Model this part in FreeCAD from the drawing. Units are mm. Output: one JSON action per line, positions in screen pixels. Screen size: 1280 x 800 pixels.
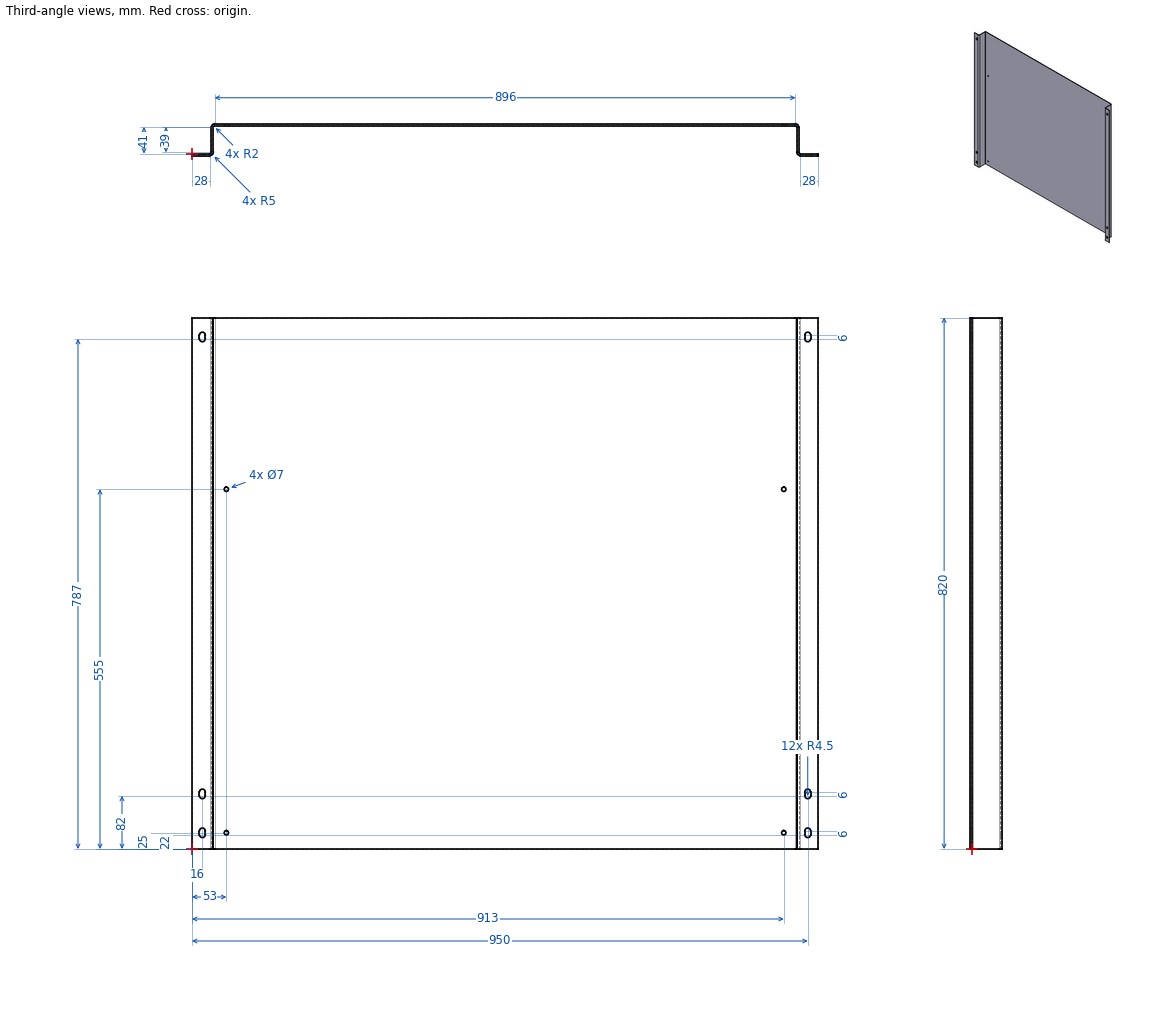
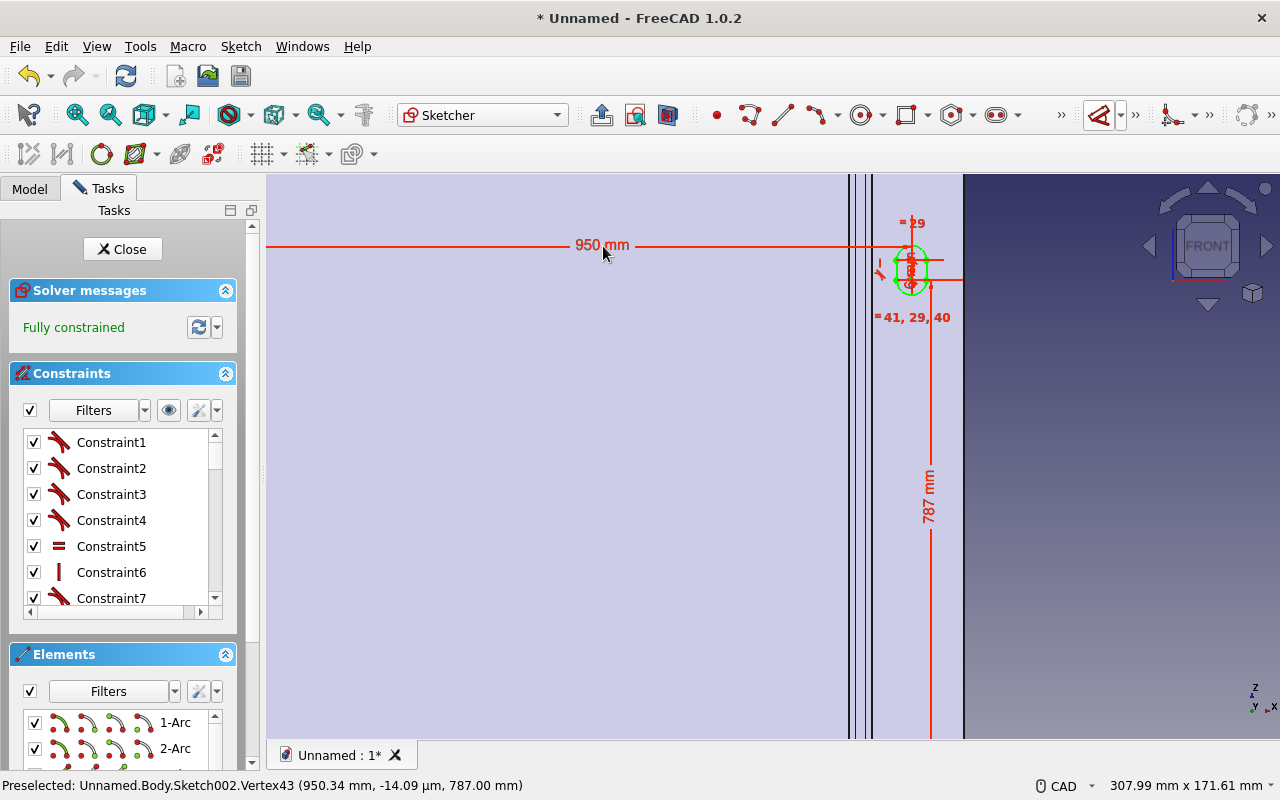
{"action": "left_click", "coordinate": [123, 249]}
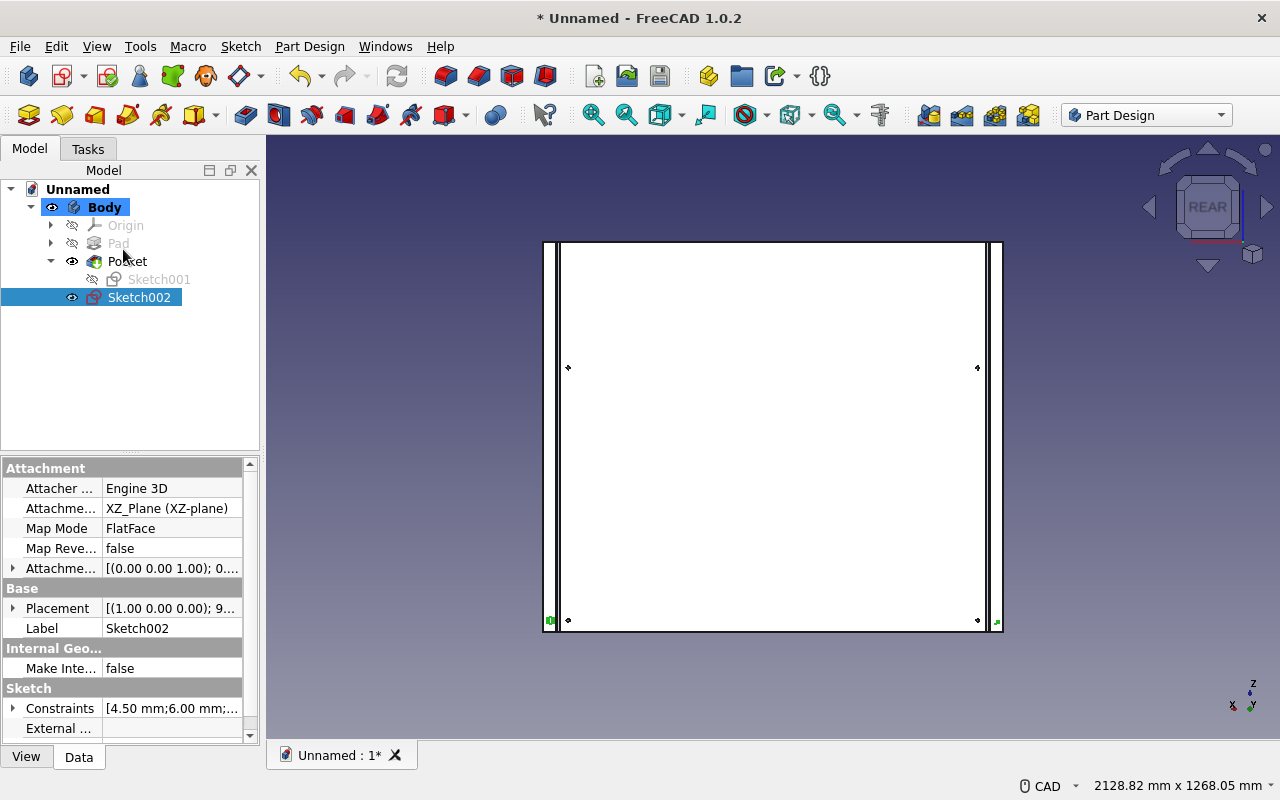
{"action": "left_click", "coordinate": [246, 116]}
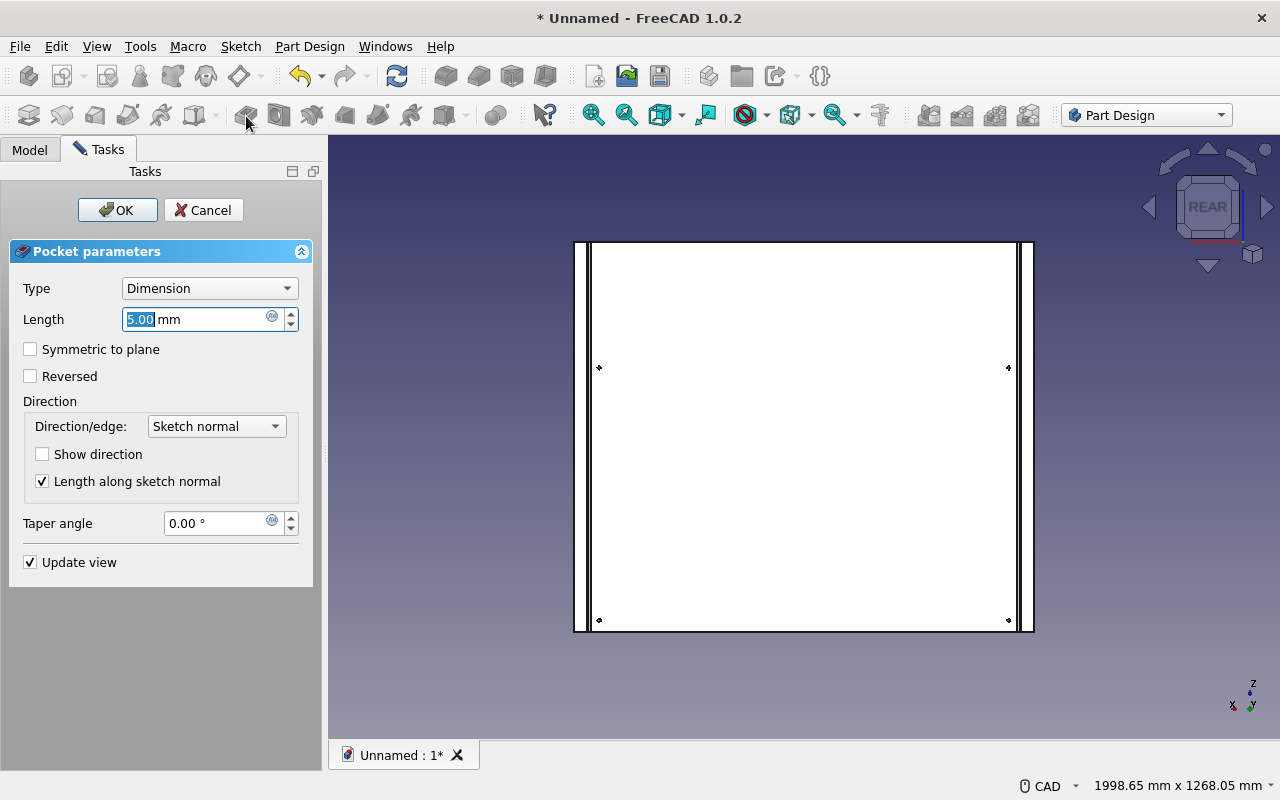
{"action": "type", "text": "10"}
{"action": "key", "text": "Tab"}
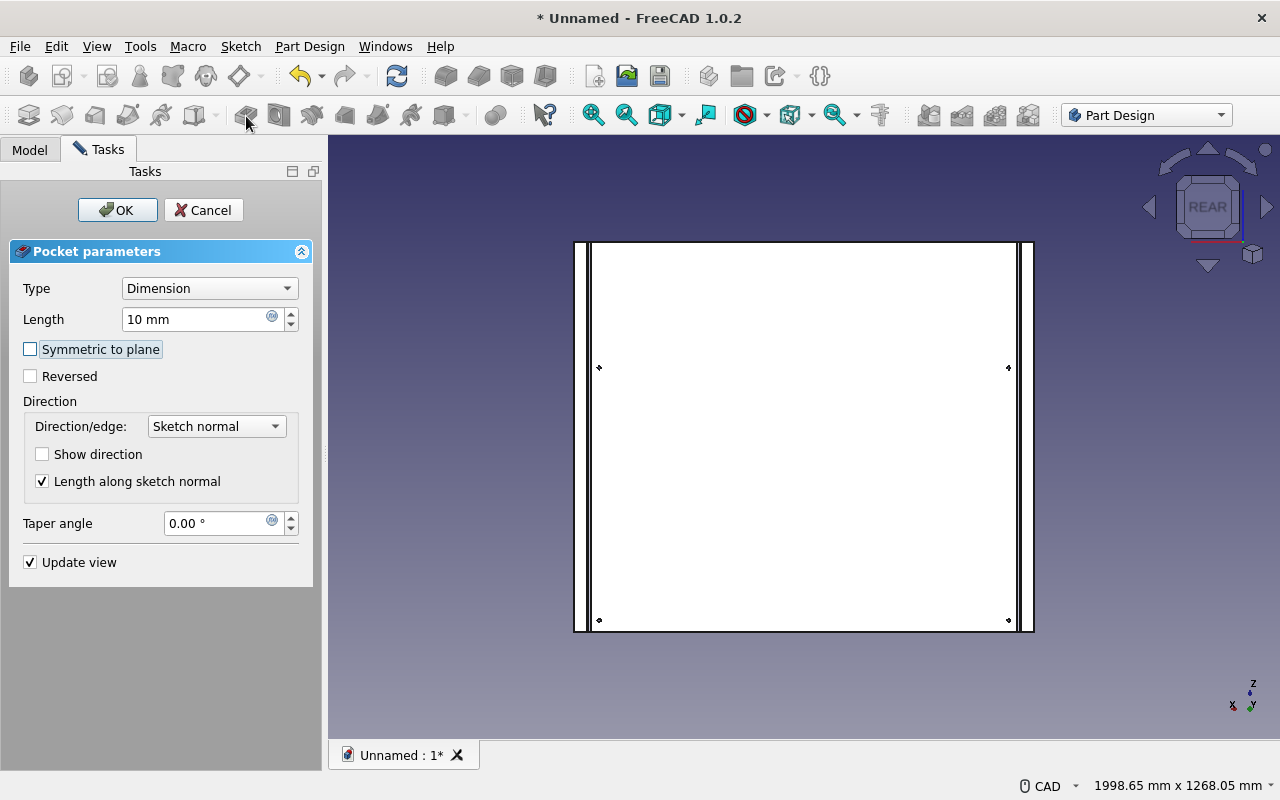
{"action": "left_click", "coordinate": [31, 376]}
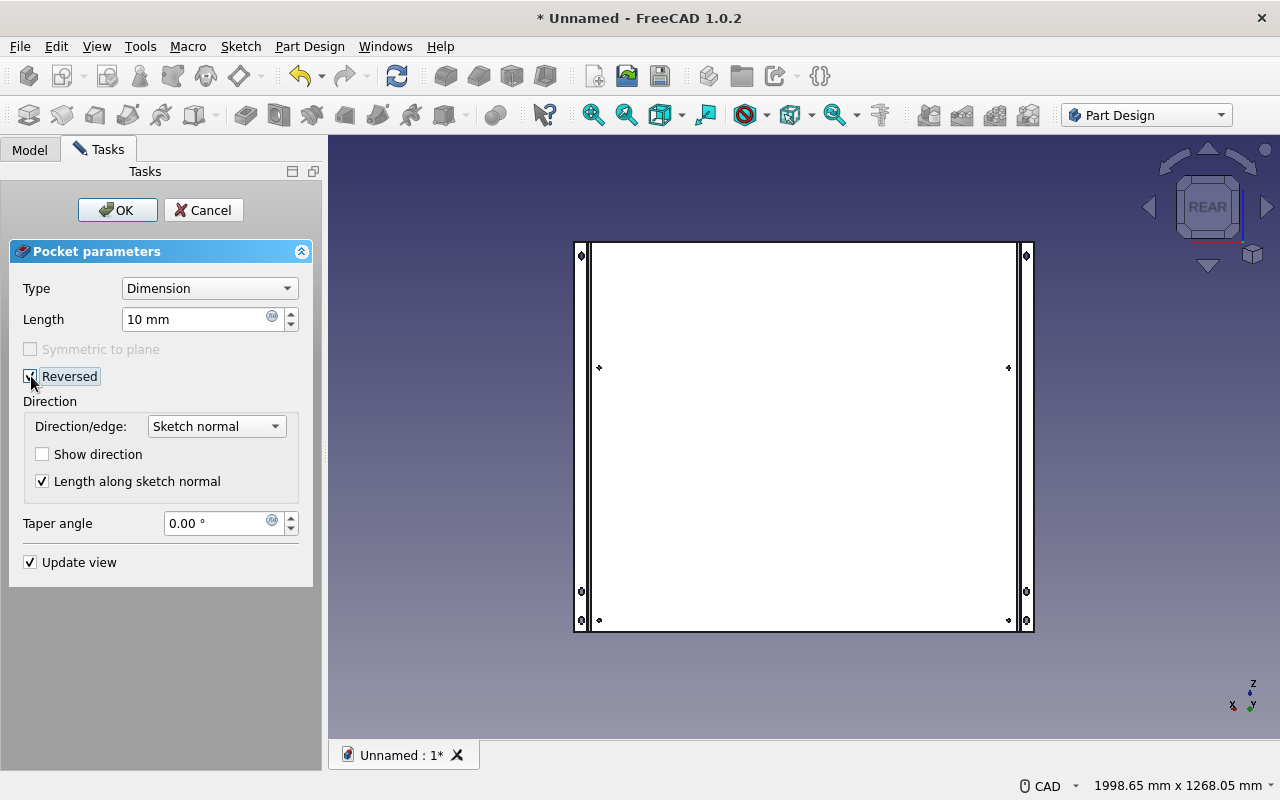
{"action": "left_click", "coordinate": [118, 210]}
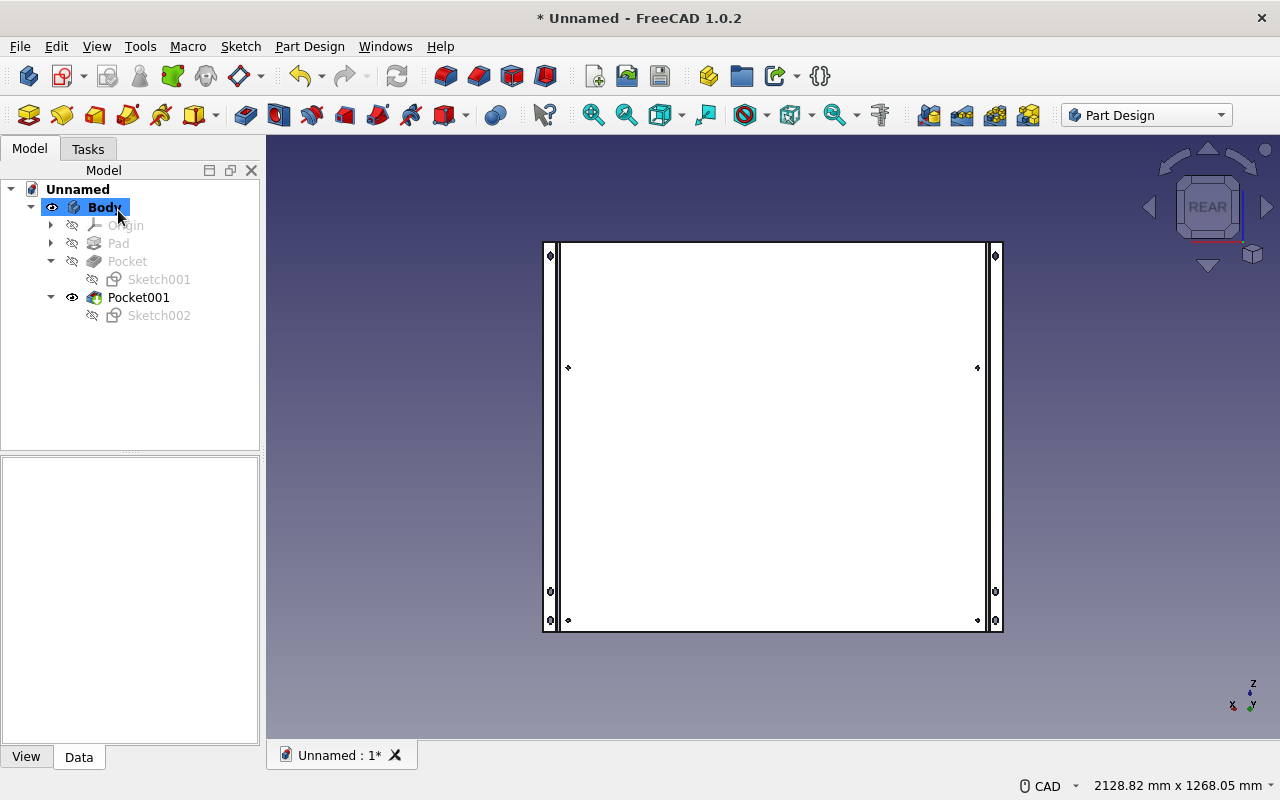
{"action": "key", "text": "0"}